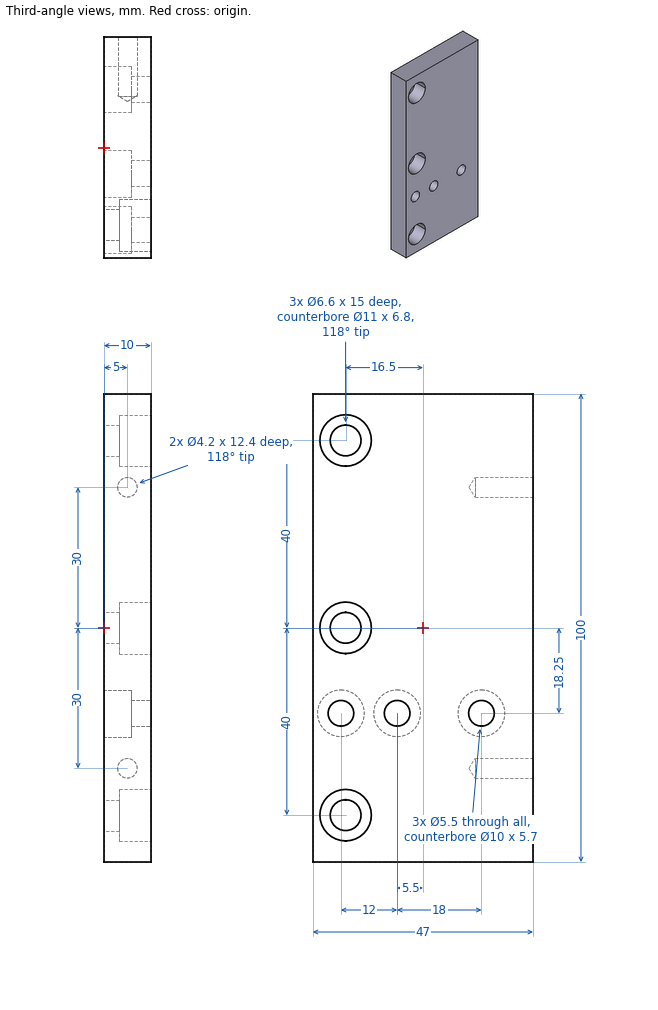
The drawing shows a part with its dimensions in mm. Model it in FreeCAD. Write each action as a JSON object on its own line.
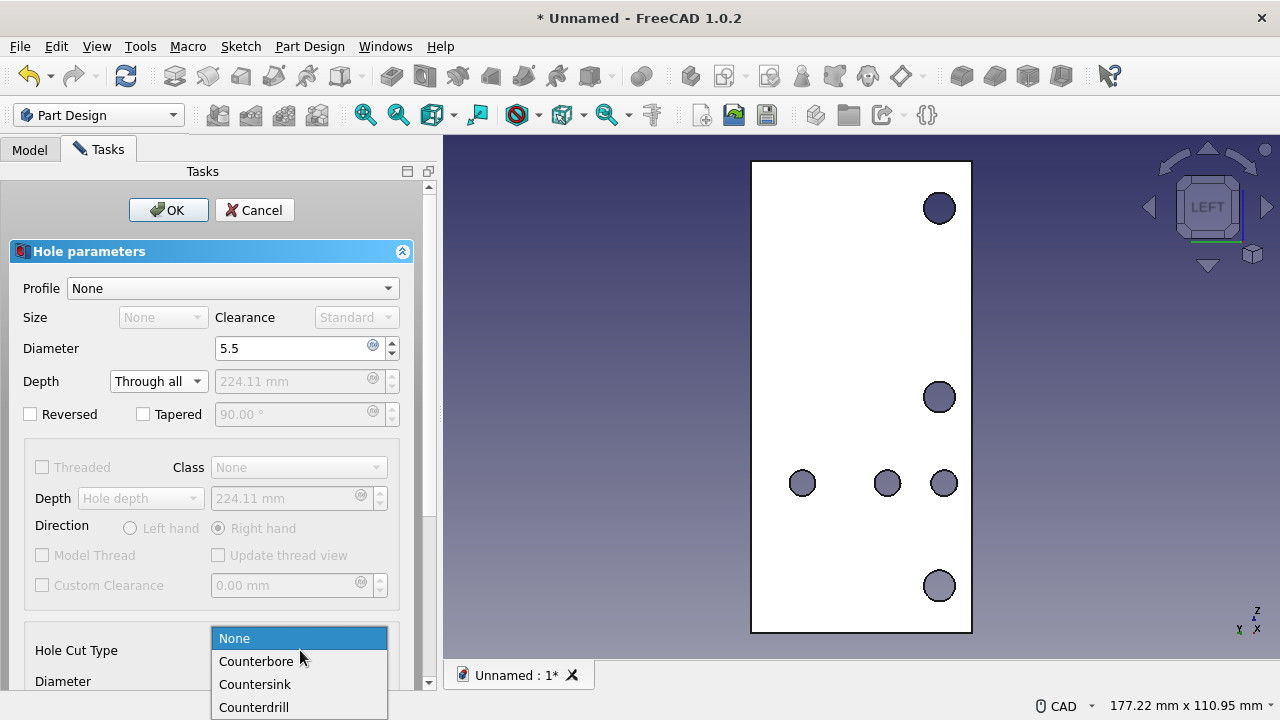
{"action": "left_click", "coordinate": [298, 662]}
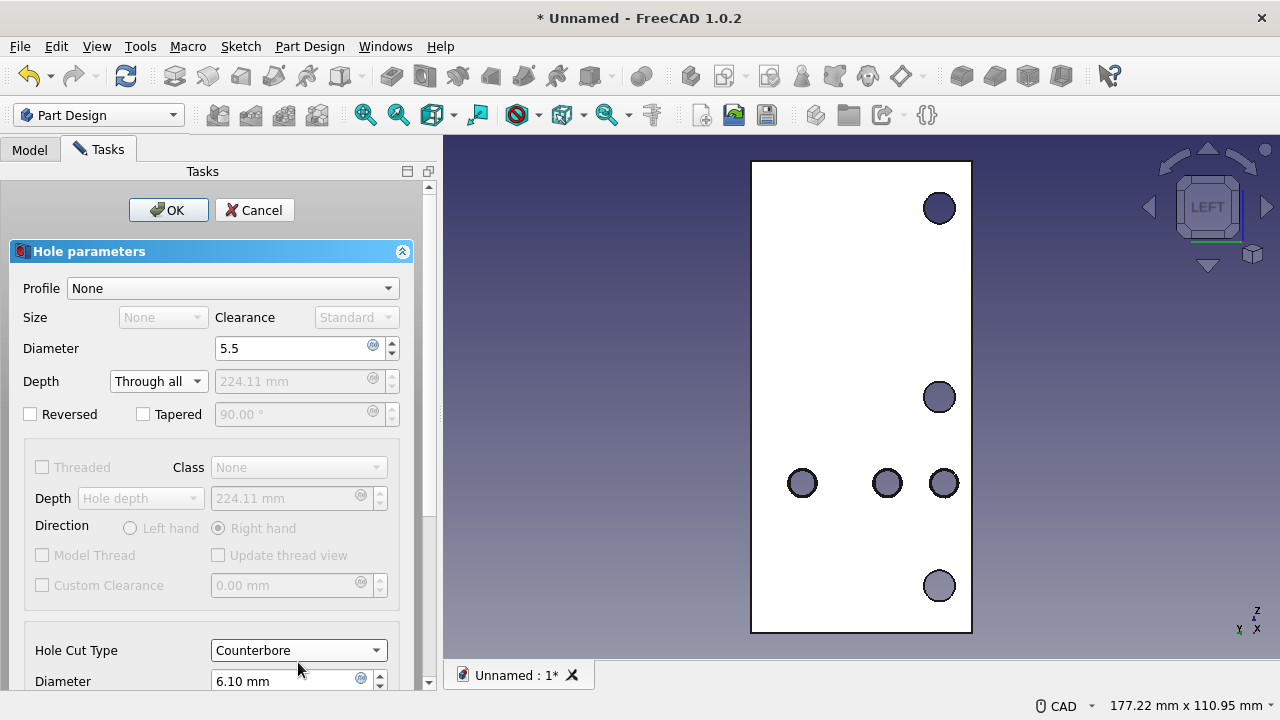
{"action": "scroll", "coordinate": [429, 436], "scroll_direction": "down", "scroll_amount": 2}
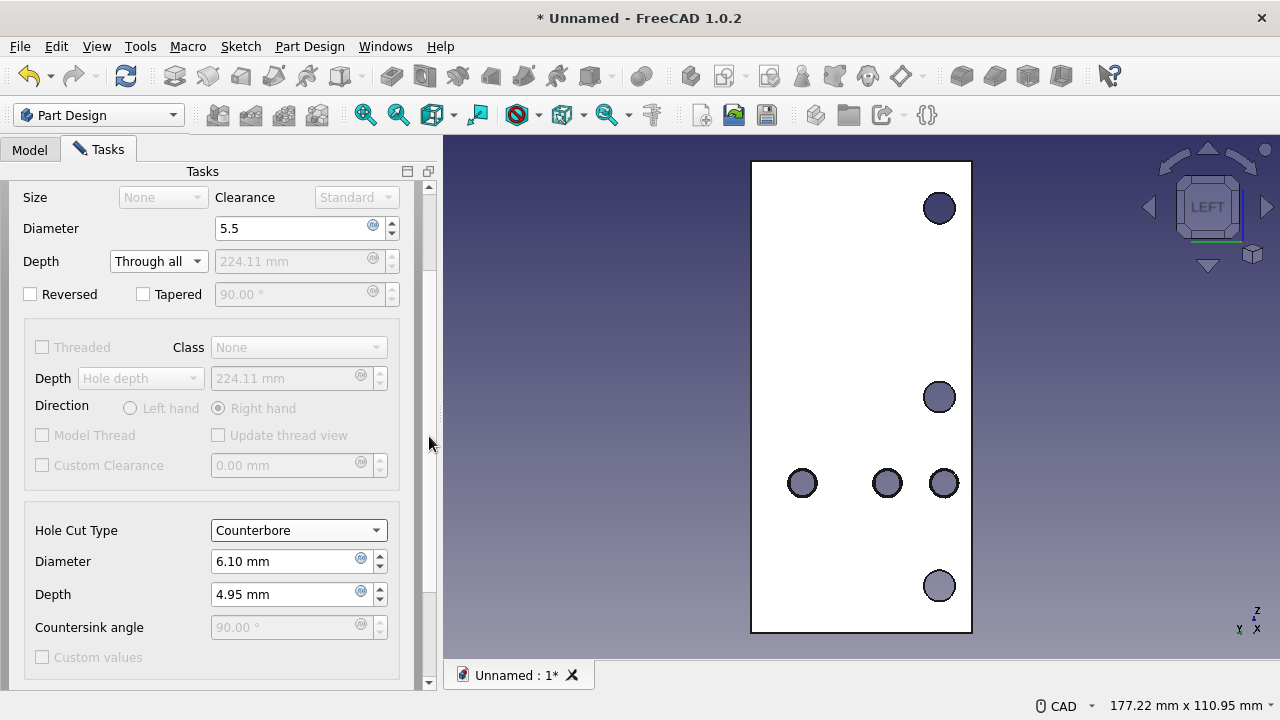
{"action": "triple_click", "coordinate": [292, 562]}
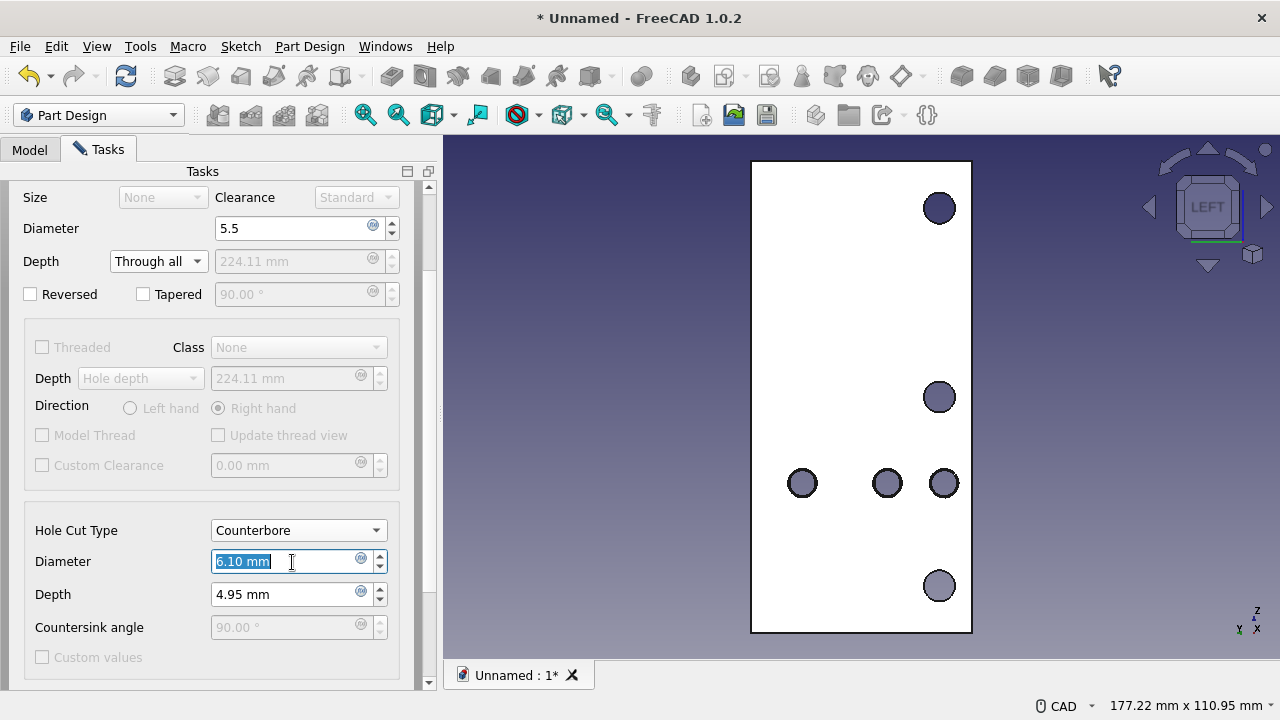
{"action": "type", "text": "10"}
{"action": "key", "text": "Tab"}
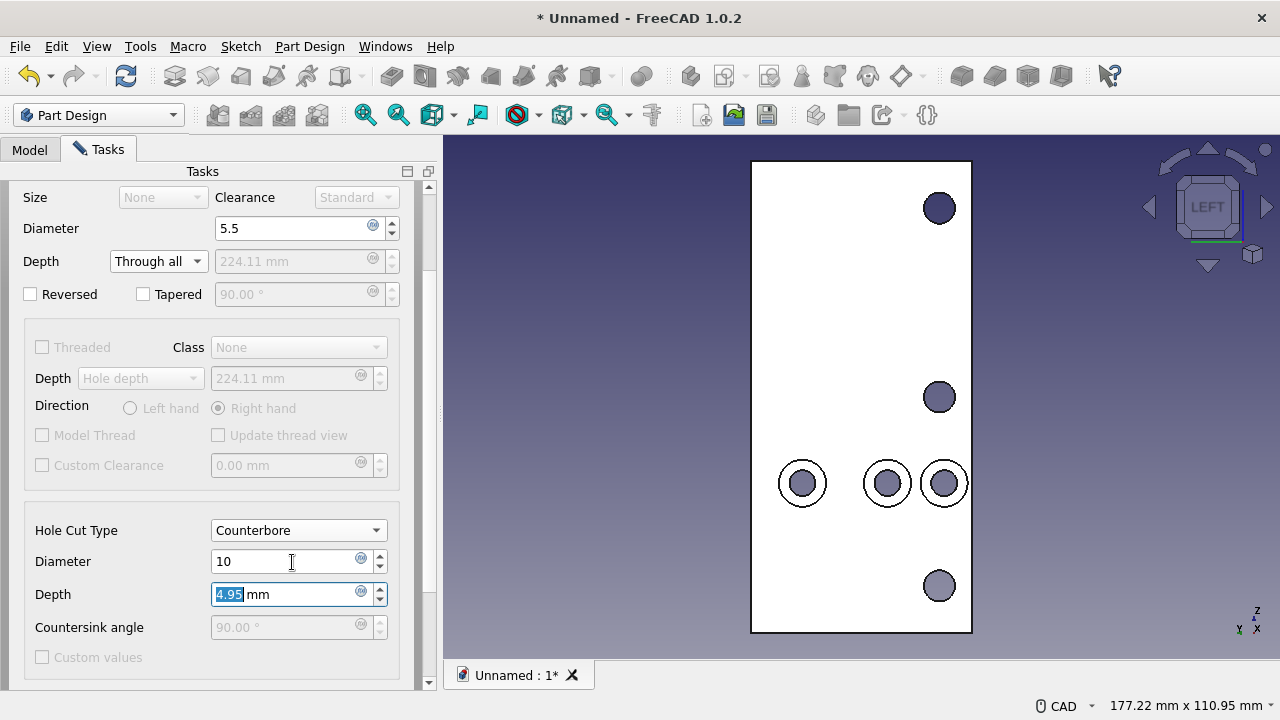
{"action": "type", "text": "5.7"}
{"action": "key", "text": "Tab"}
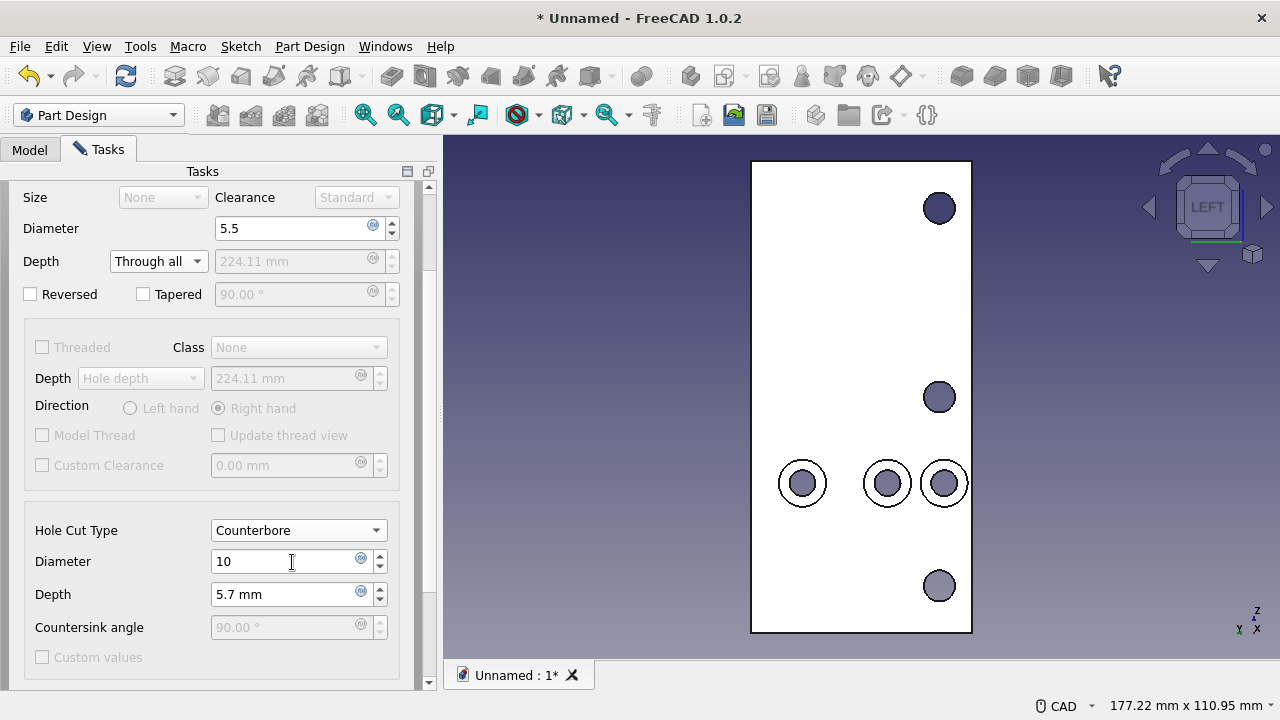
{"action": "scroll", "coordinate": [429, 436], "scroll_direction": "up", "scroll_amount": 3}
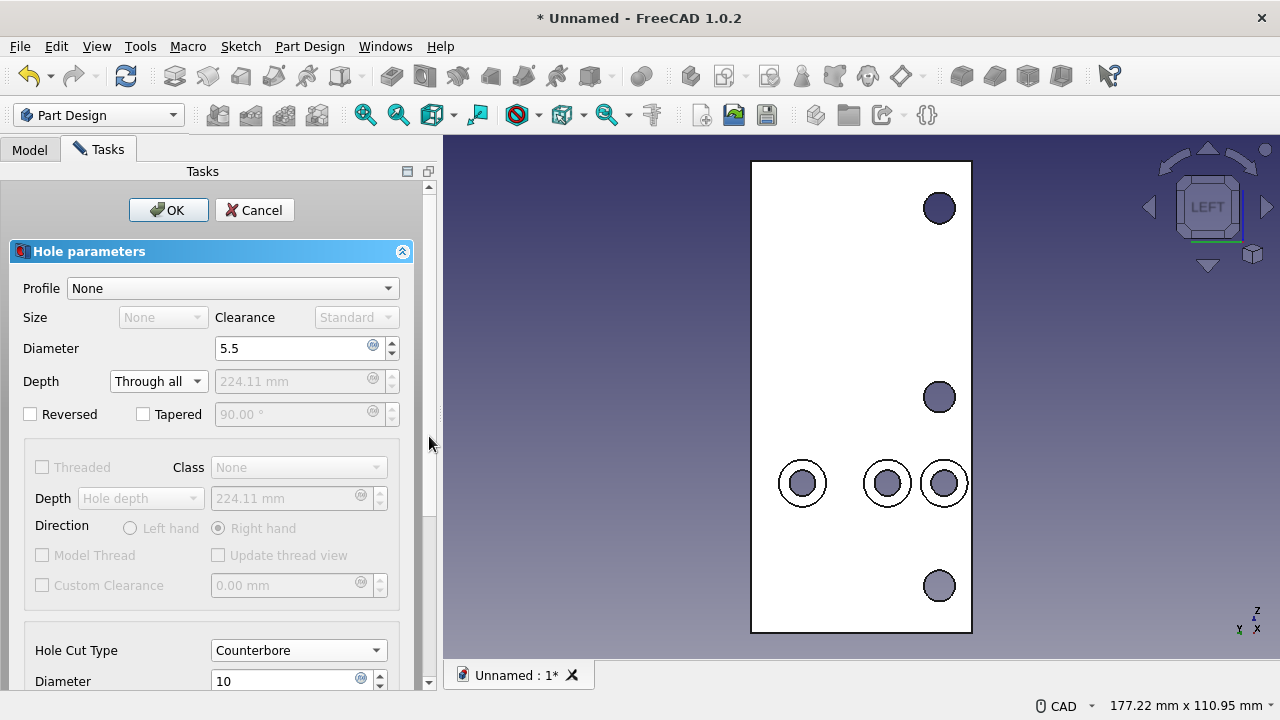
{"action": "left_click", "coordinate": [169, 210]}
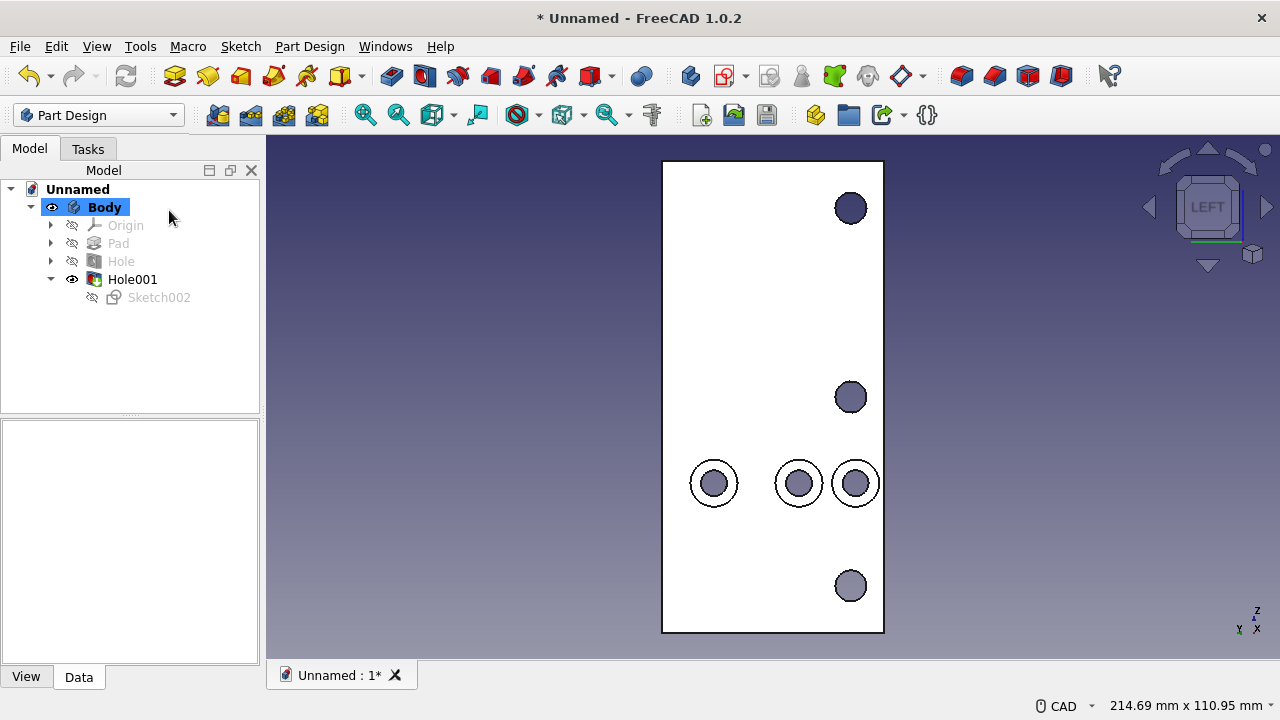
{"action": "key", "text": "4"}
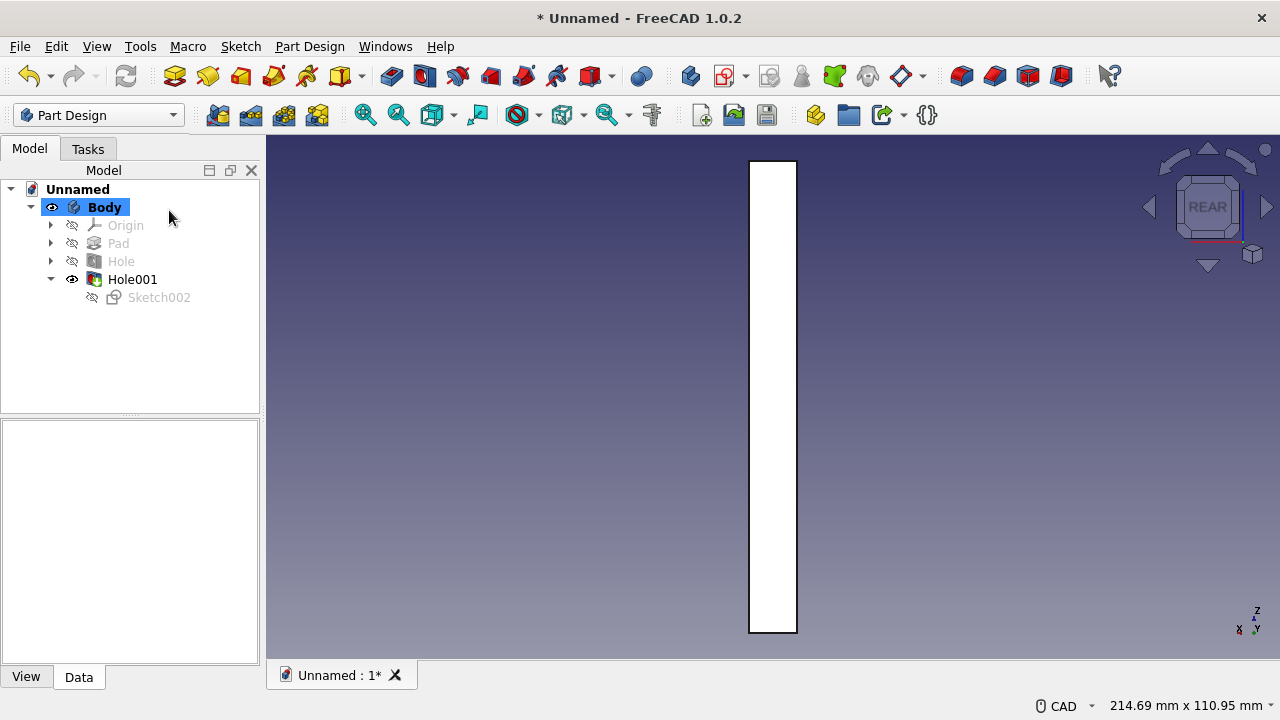
{"action": "left_click", "coordinate": [773, 396]}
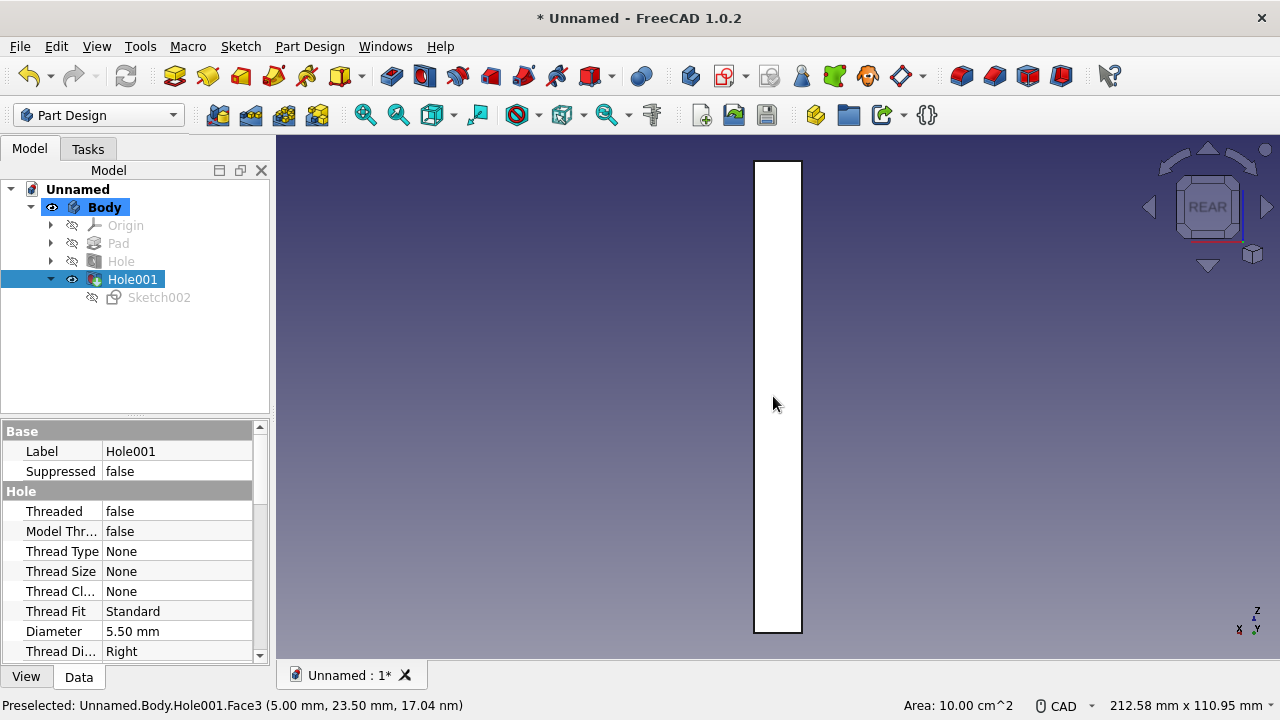
{"action": "left_click", "coordinate": [724, 76]}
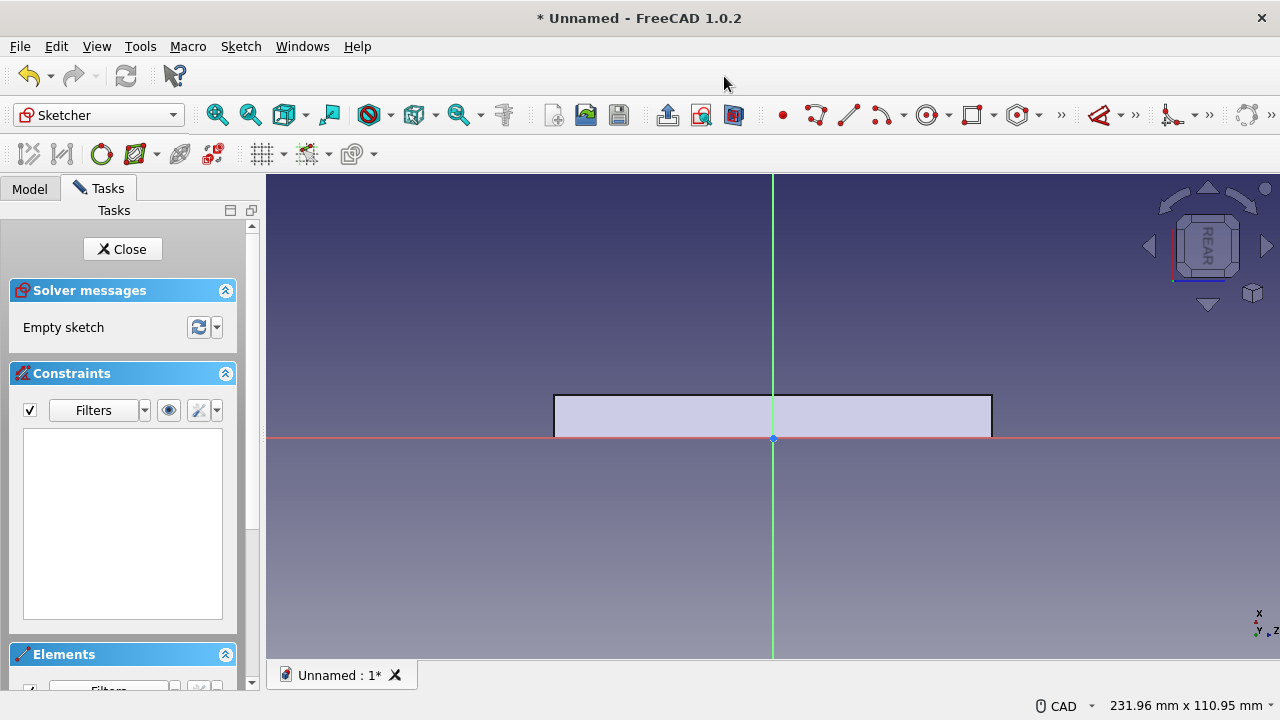
{"action": "scroll", "coordinate": [829, 428], "scroll_direction": "up", "scroll_amount": 4}